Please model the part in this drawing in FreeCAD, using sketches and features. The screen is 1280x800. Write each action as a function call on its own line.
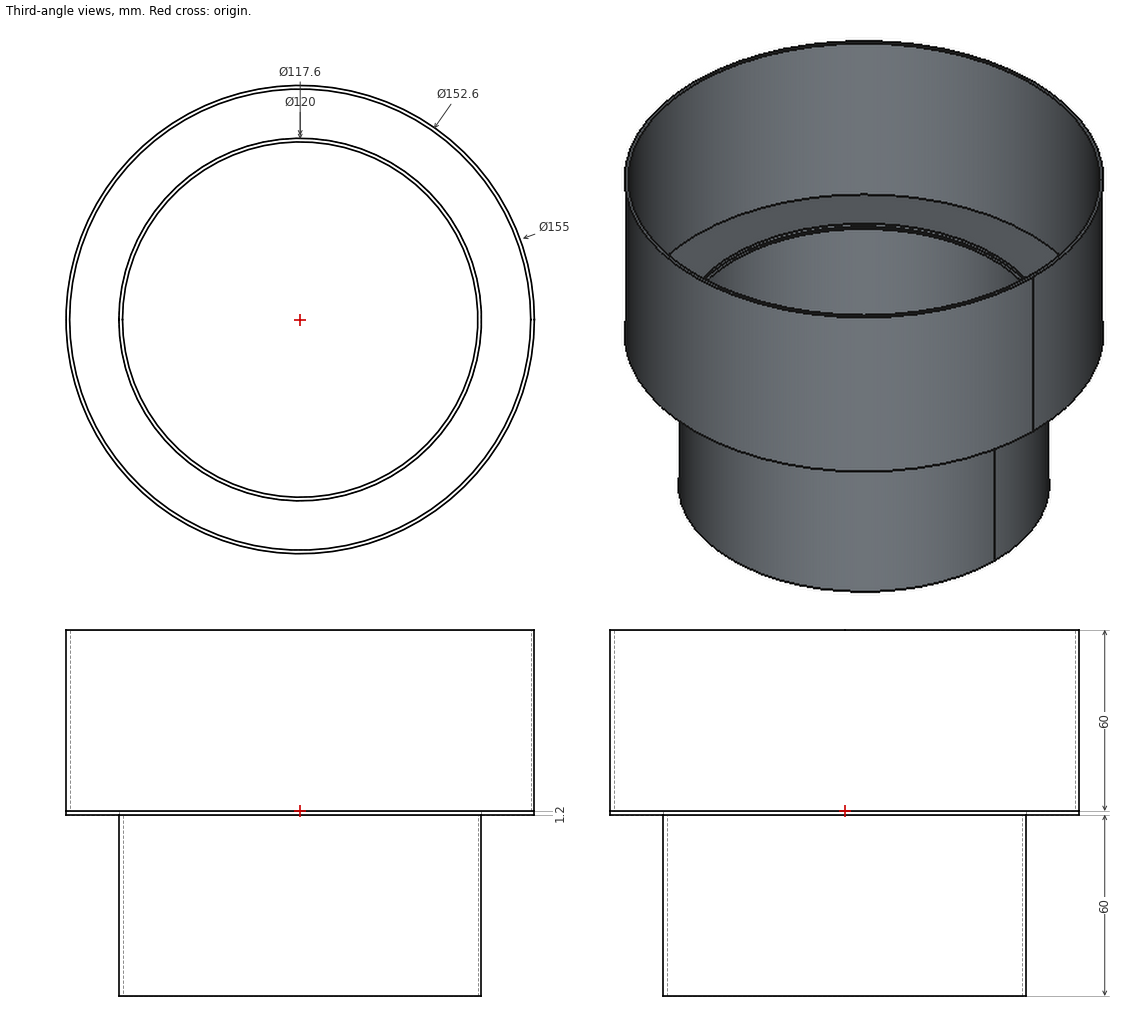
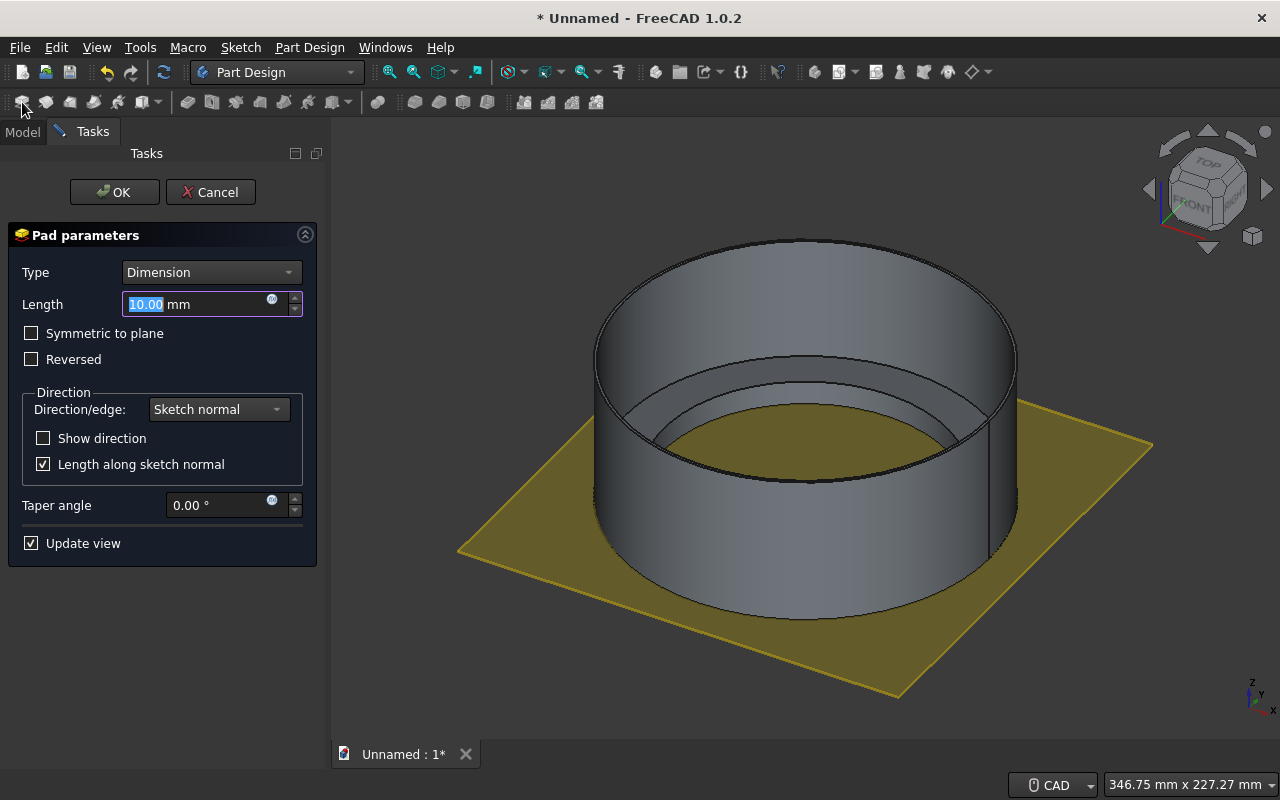
text(1.2)
key(Tab)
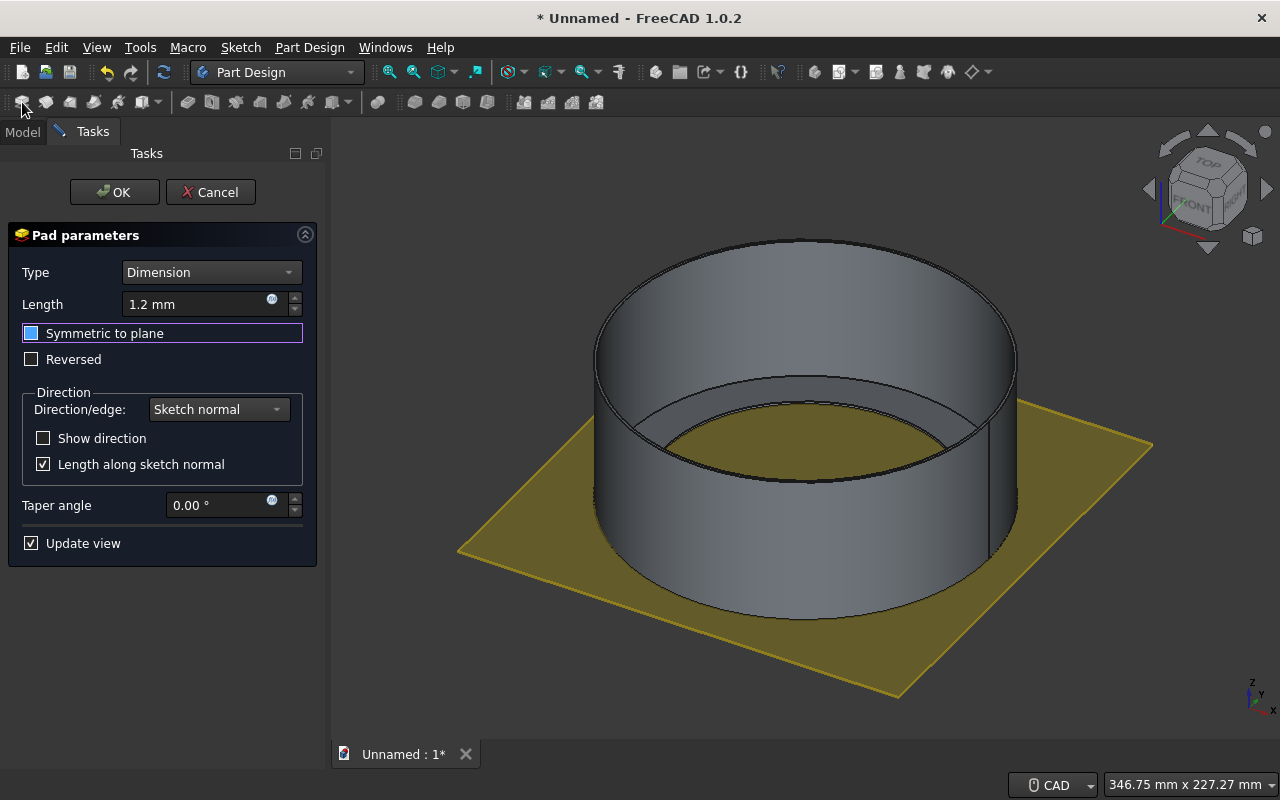
click(115, 192)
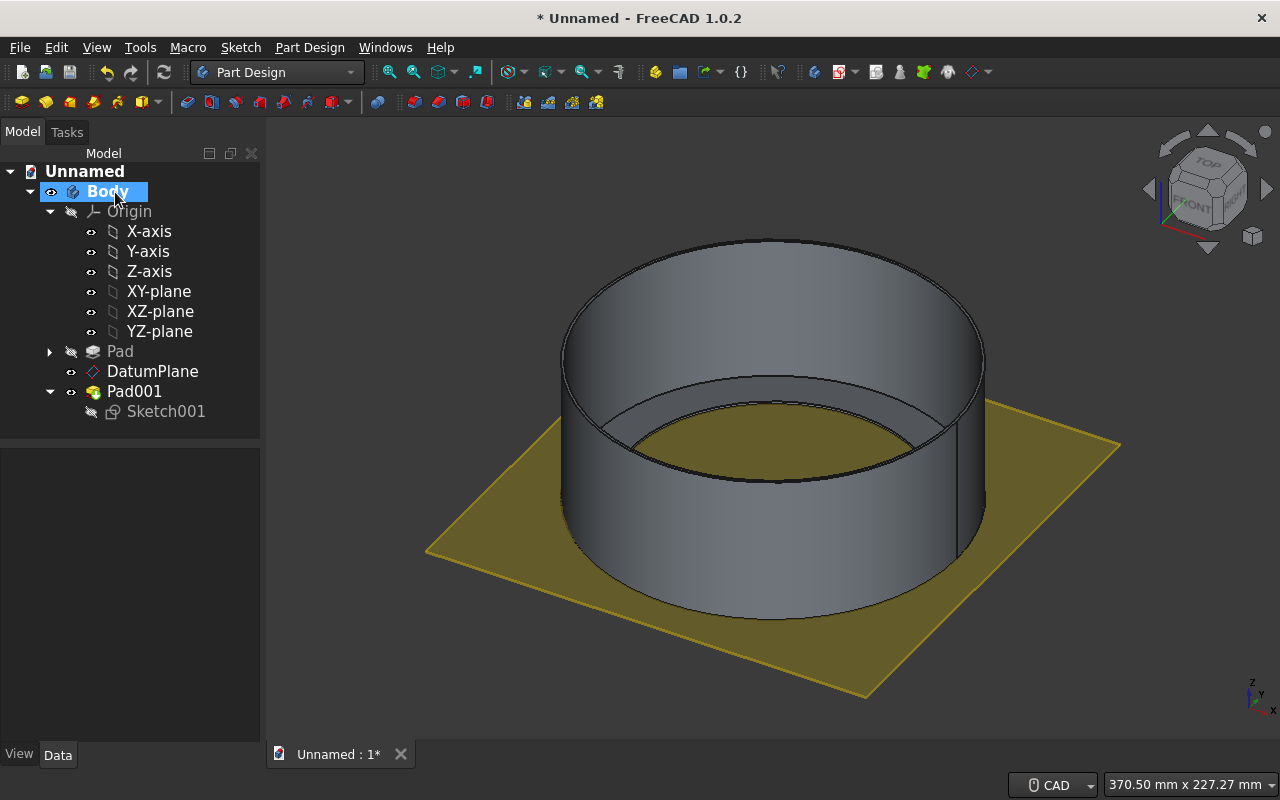
click(116, 372)
key(space)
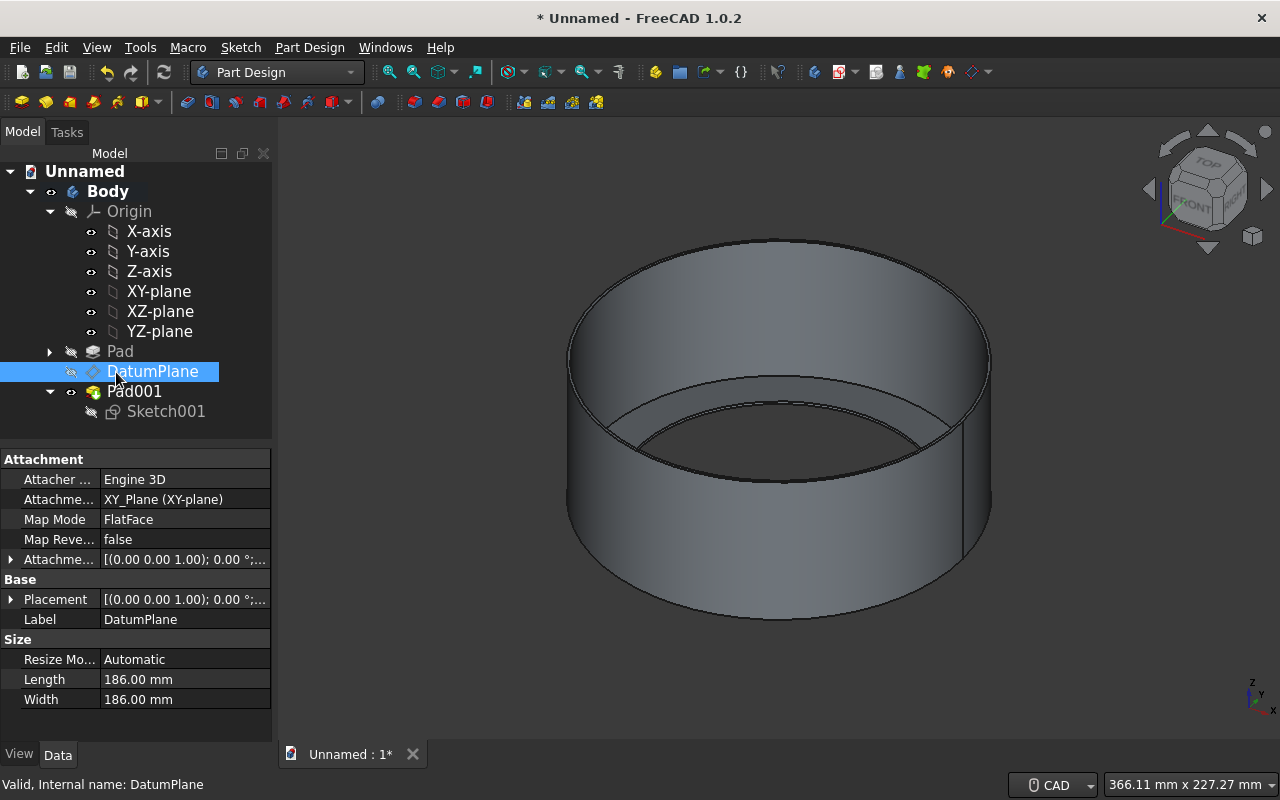
click(318, 699)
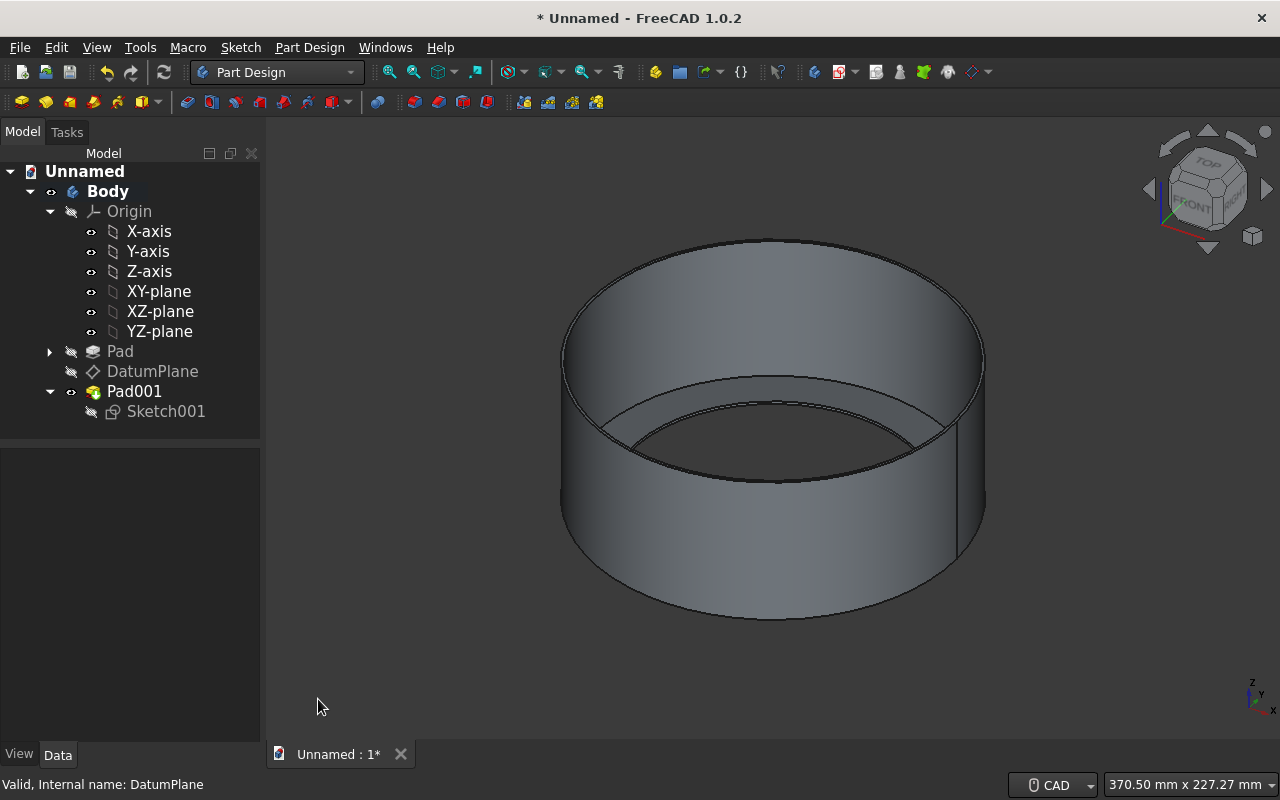
click(816, 72)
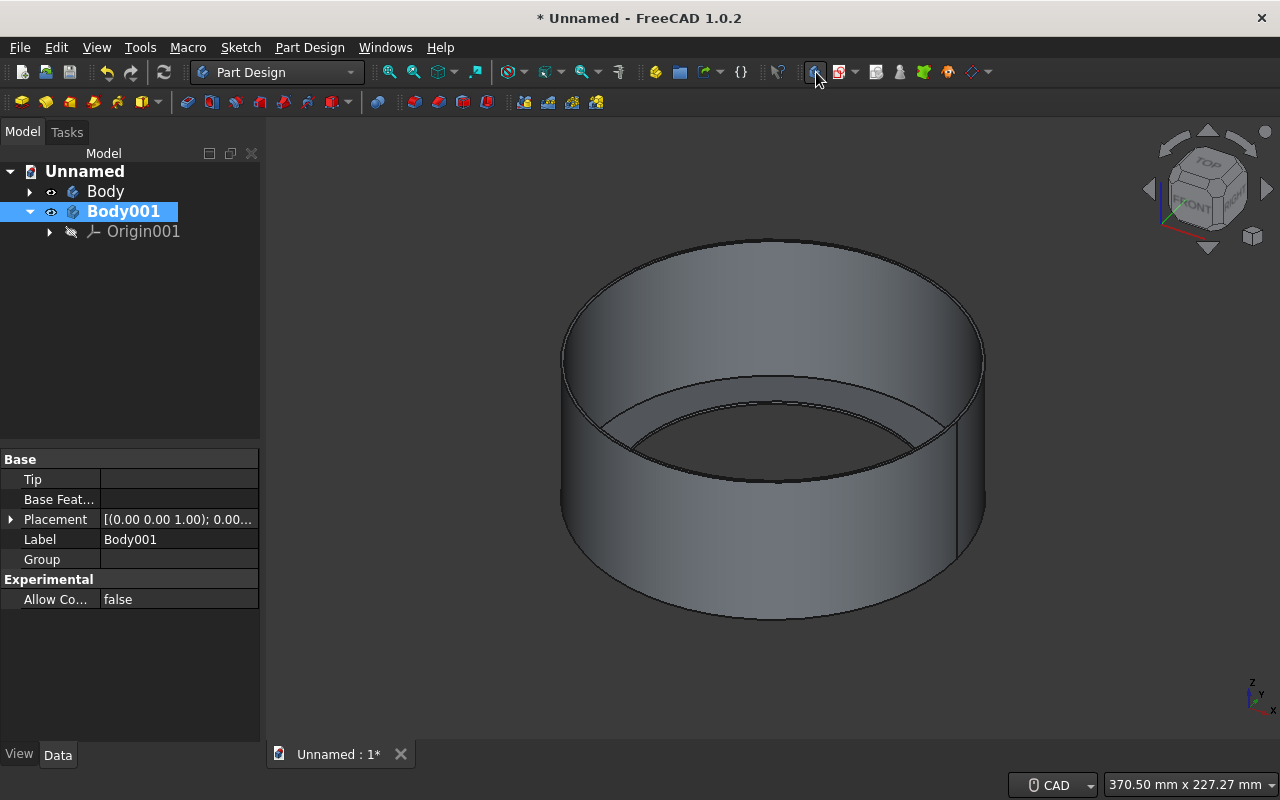
click(50, 232)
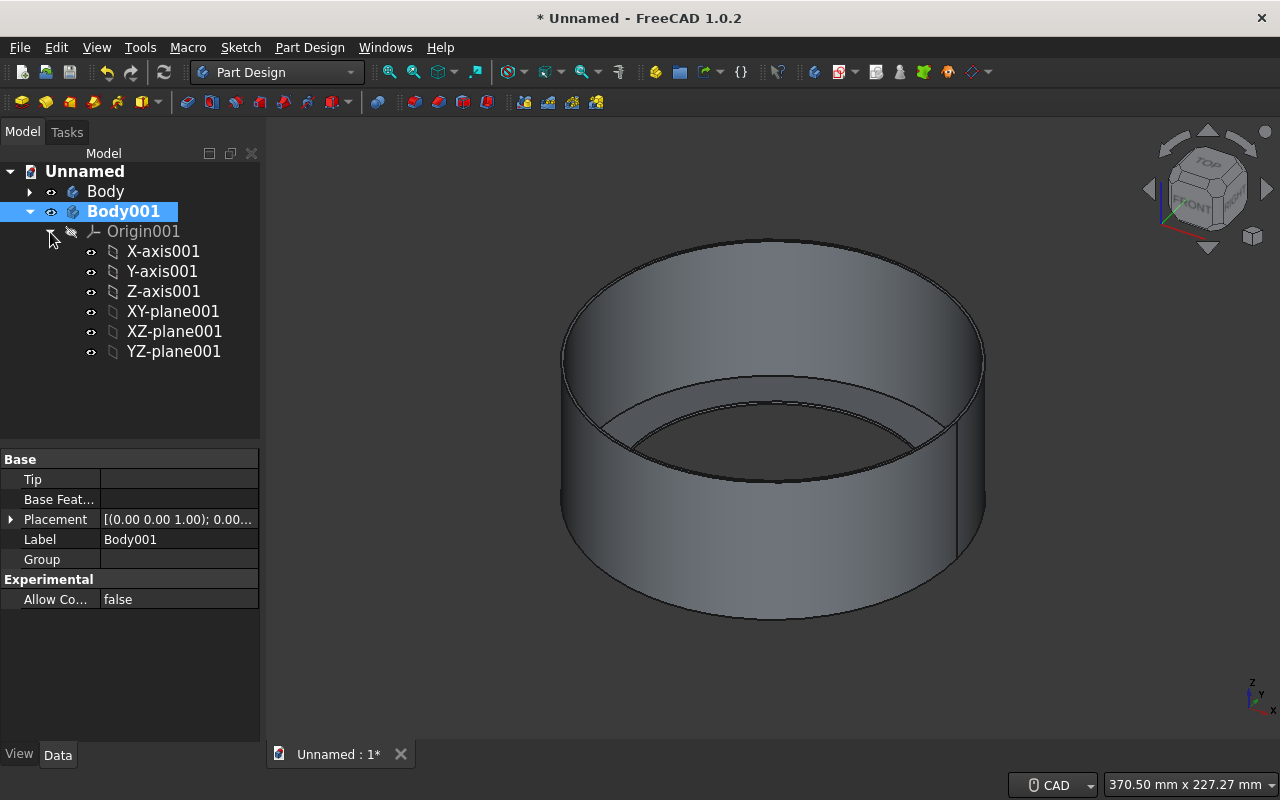
click(136, 312)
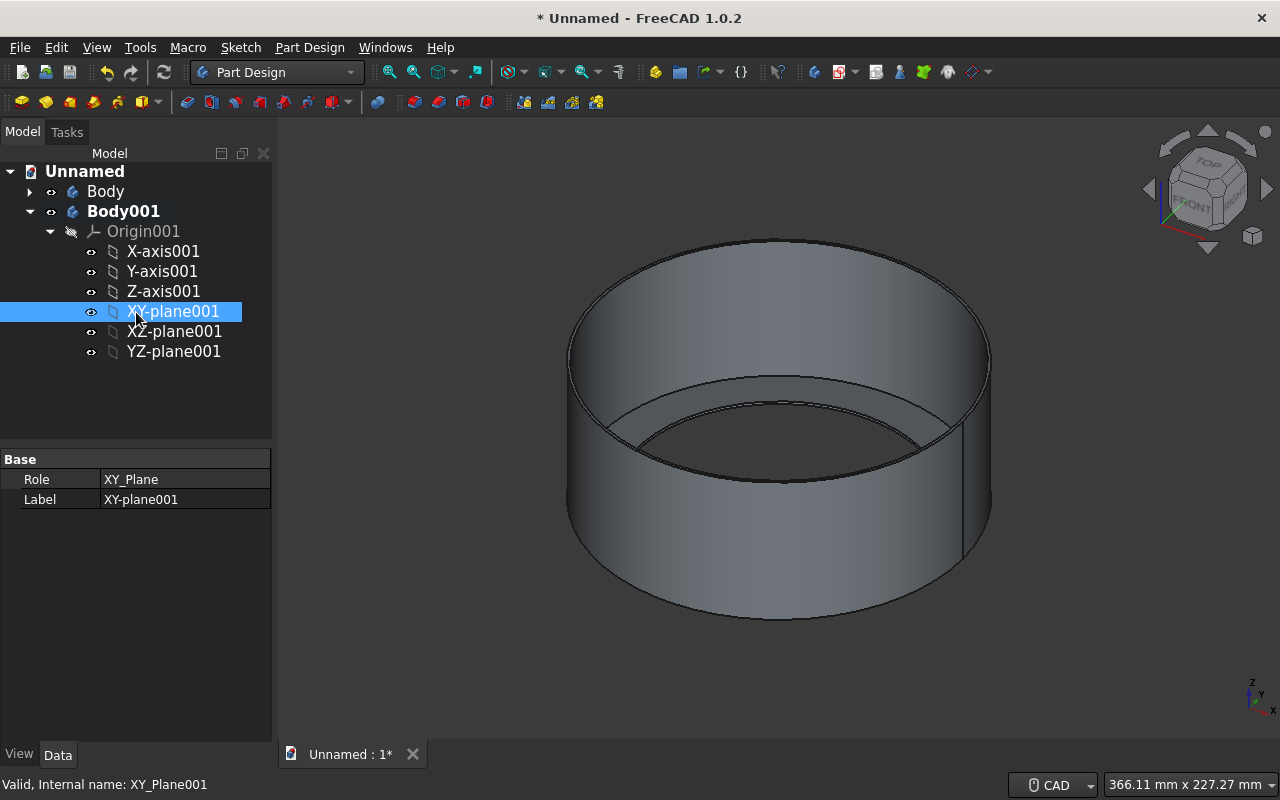
click(972, 72)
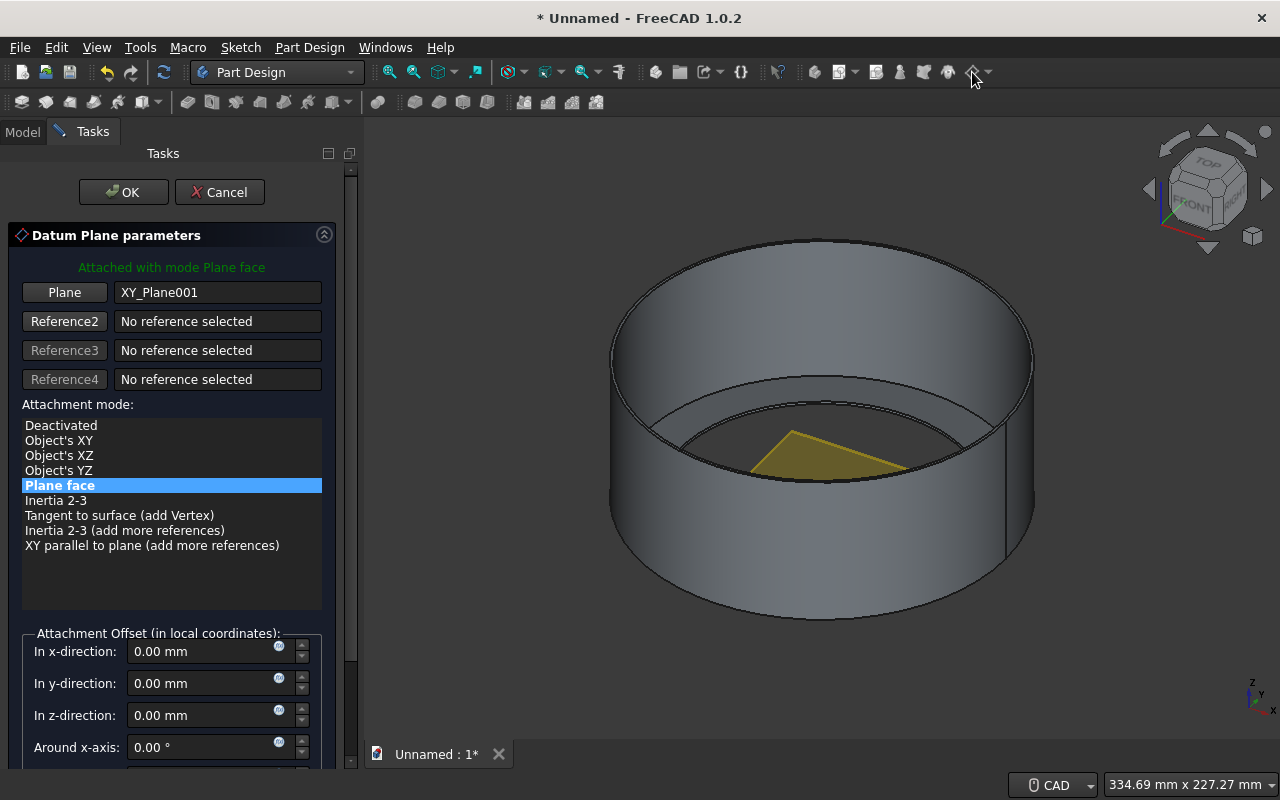
triple_click(210, 715)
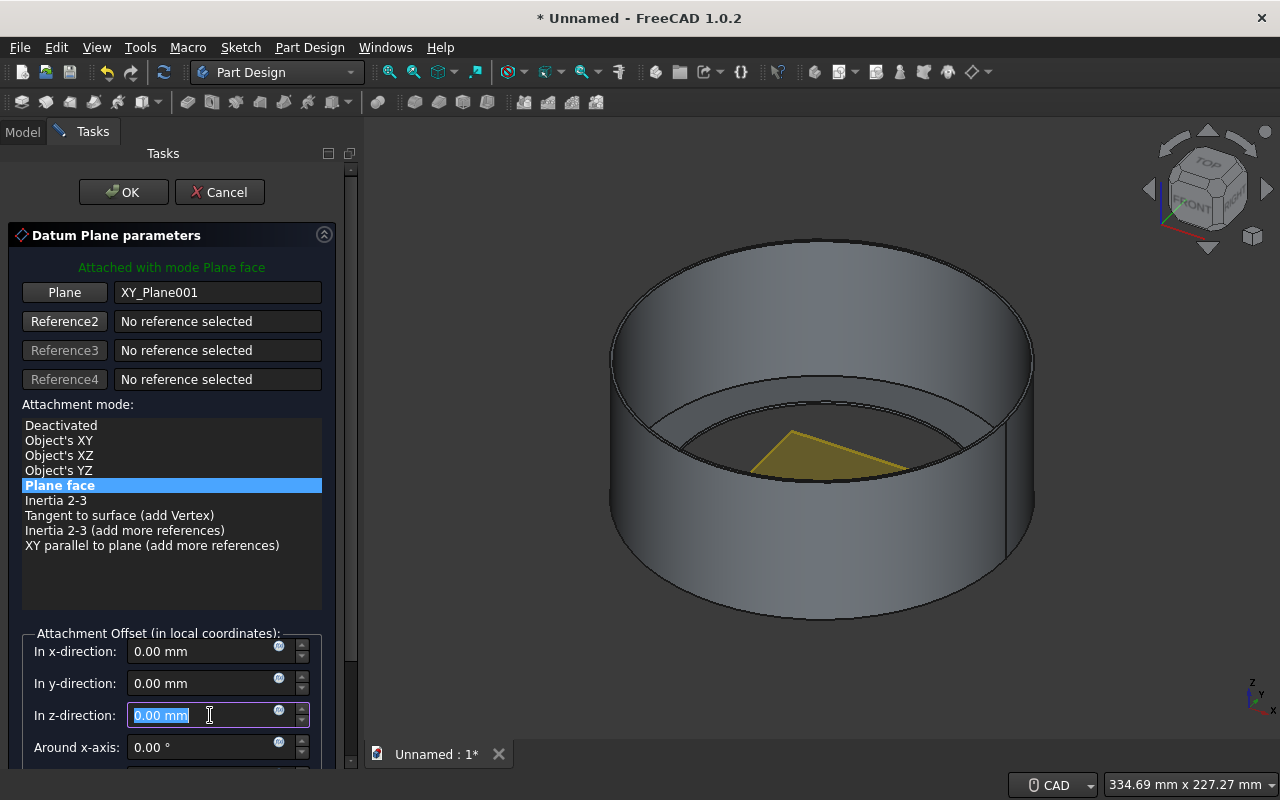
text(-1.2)
key(Tab)